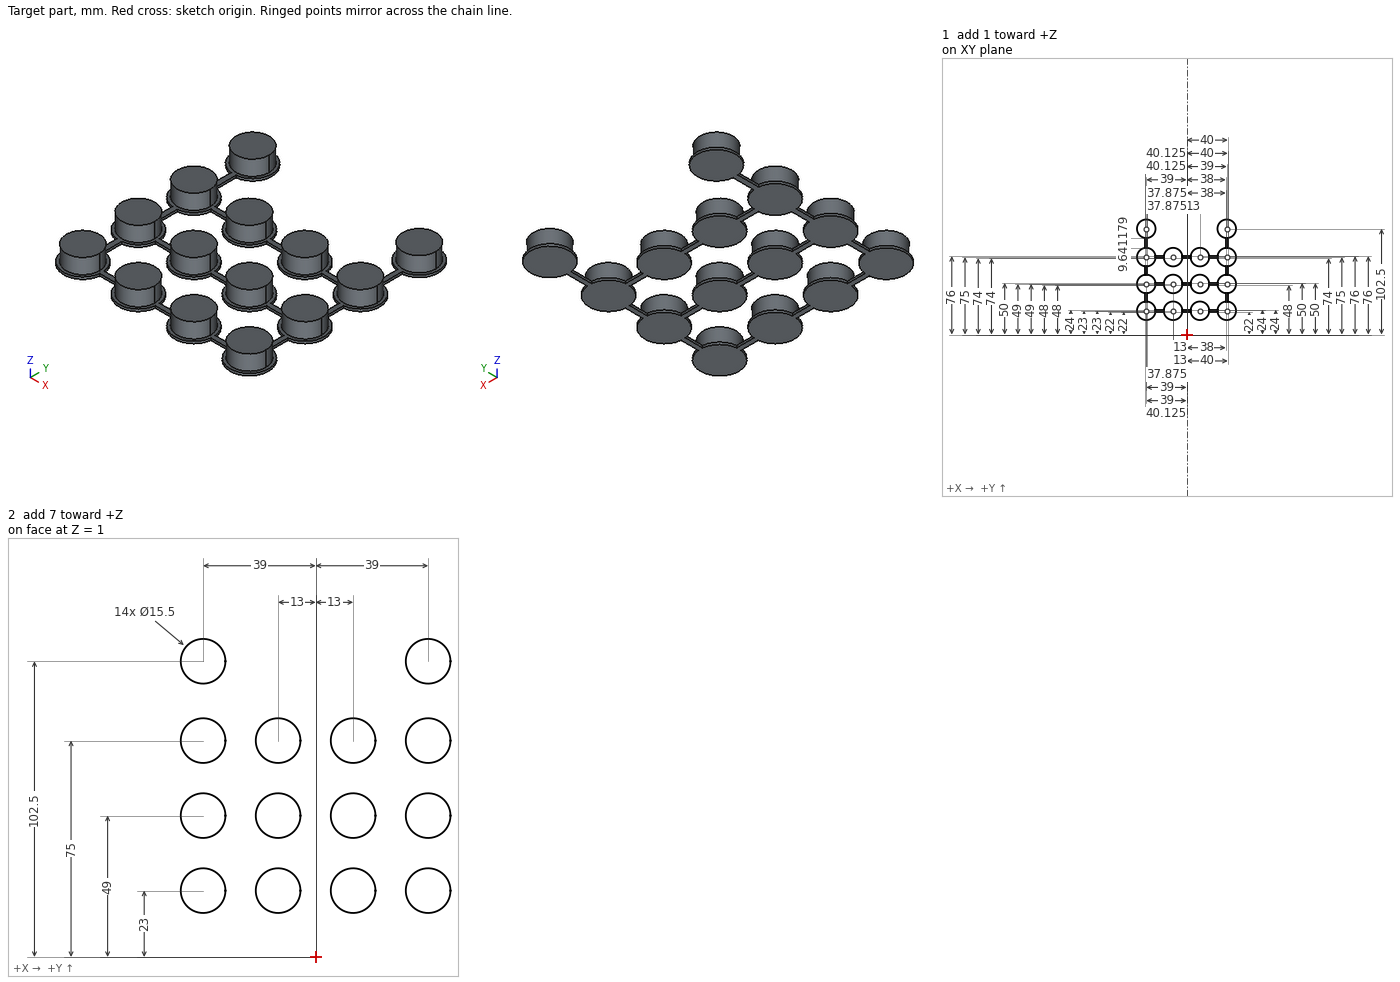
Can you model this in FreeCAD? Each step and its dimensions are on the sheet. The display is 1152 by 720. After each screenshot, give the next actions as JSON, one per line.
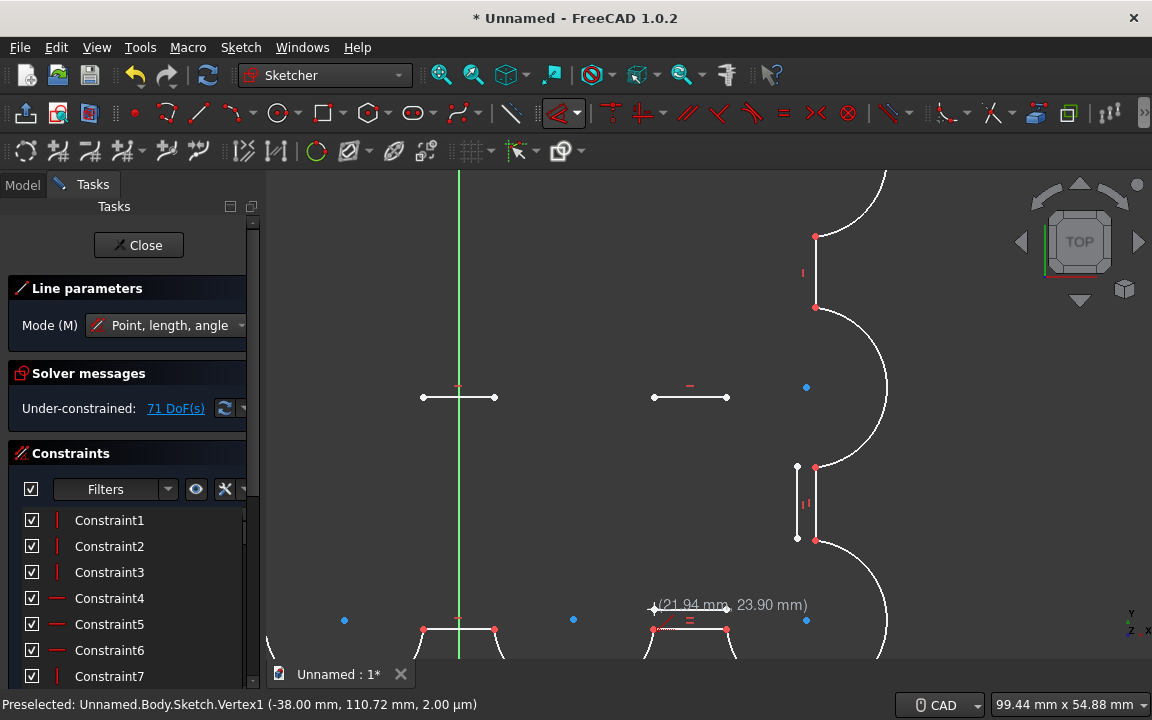
{"action": "left_click", "coordinate": [495, 609]}
{"action": "left_click", "coordinate": [422, 609]}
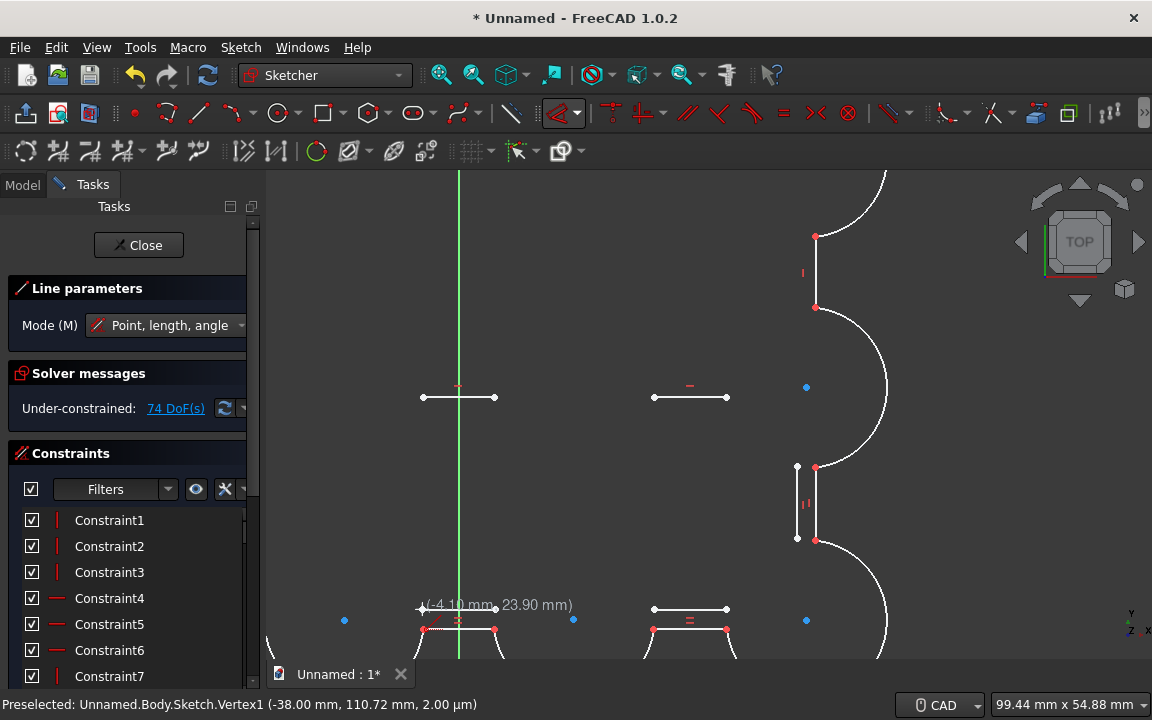
{"action": "scroll", "coordinate": [719, 453], "scroll_direction": "down", "scroll_amount": 6}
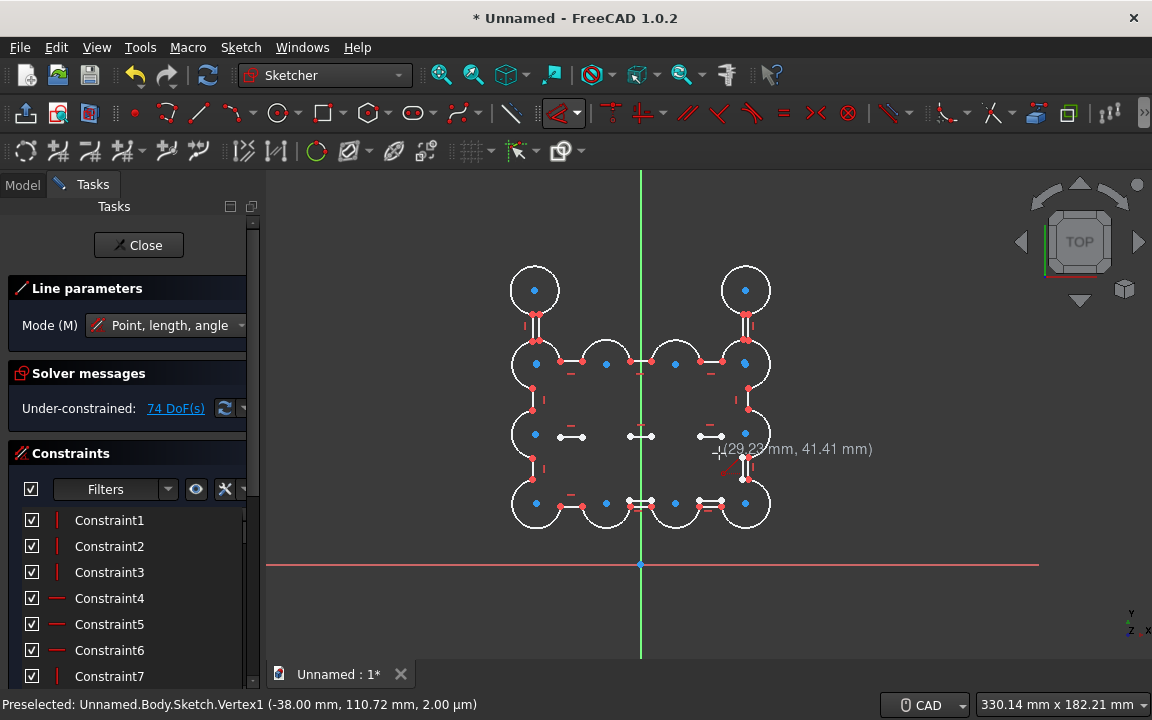
{"action": "scroll", "coordinate": [582, 500], "scroll_direction": "up", "scroll_amount": 6}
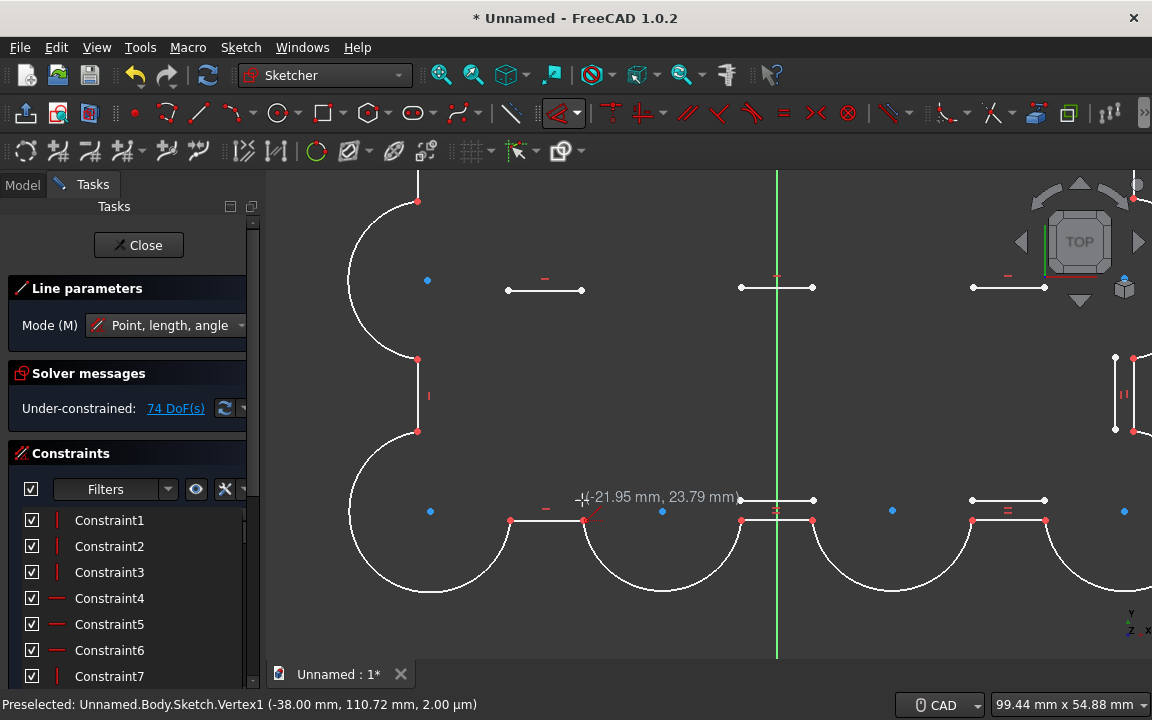
{"action": "left_click", "coordinate": [581, 500]}
{"action": "left_click", "coordinate": [509, 500]}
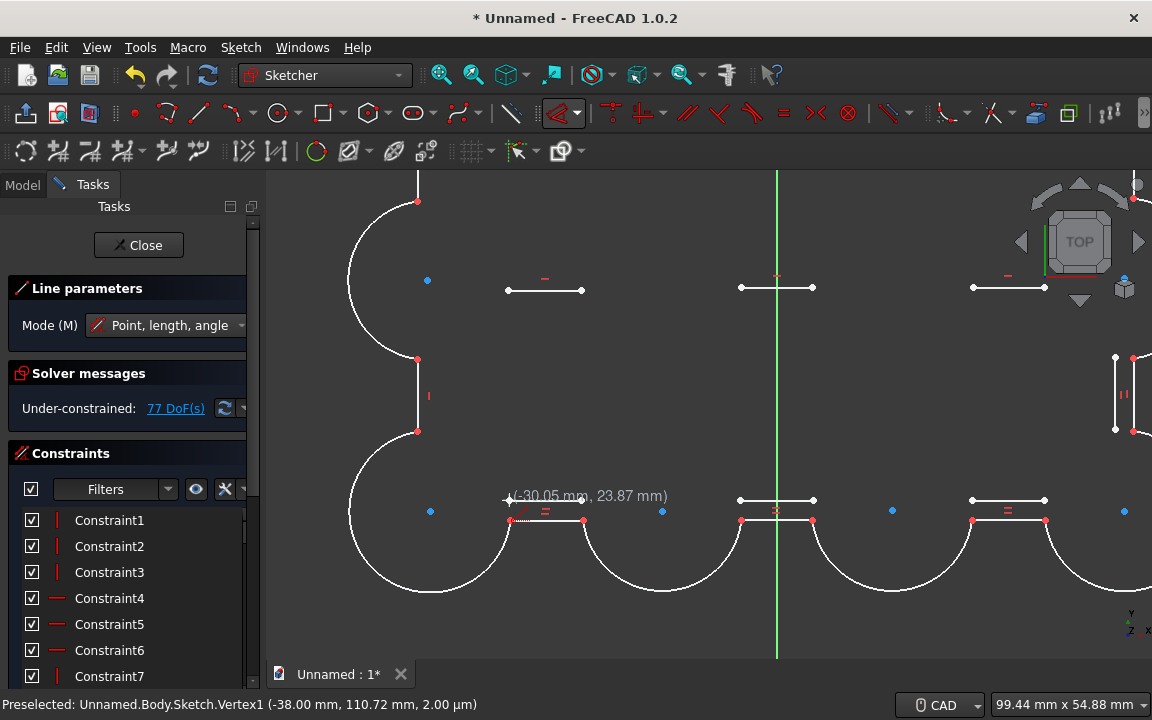
{"action": "left_click", "coordinate": [439, 429]}
{"action": "left_click", "coordinate": [439, 357]}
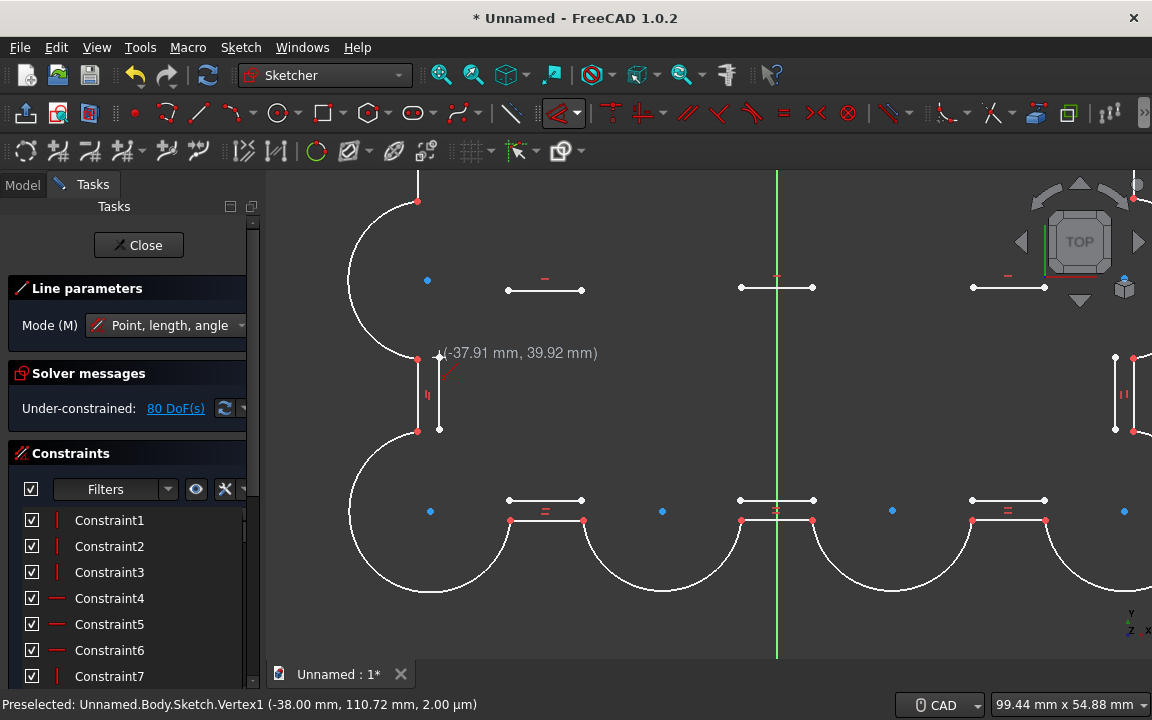
{"action": "left_click", "coordinate": [232, 114]}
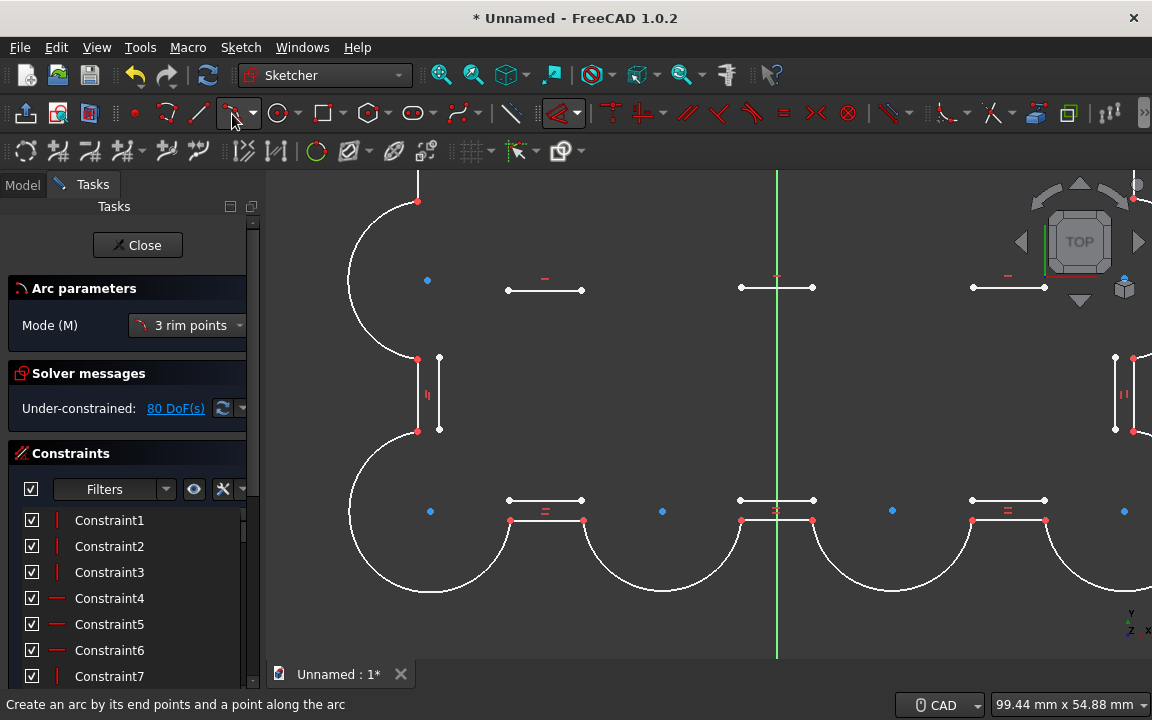
{"action": "left_click", "coordinate": [582, 291]}
{"action": "left_click", "coordinate": [742, 288]}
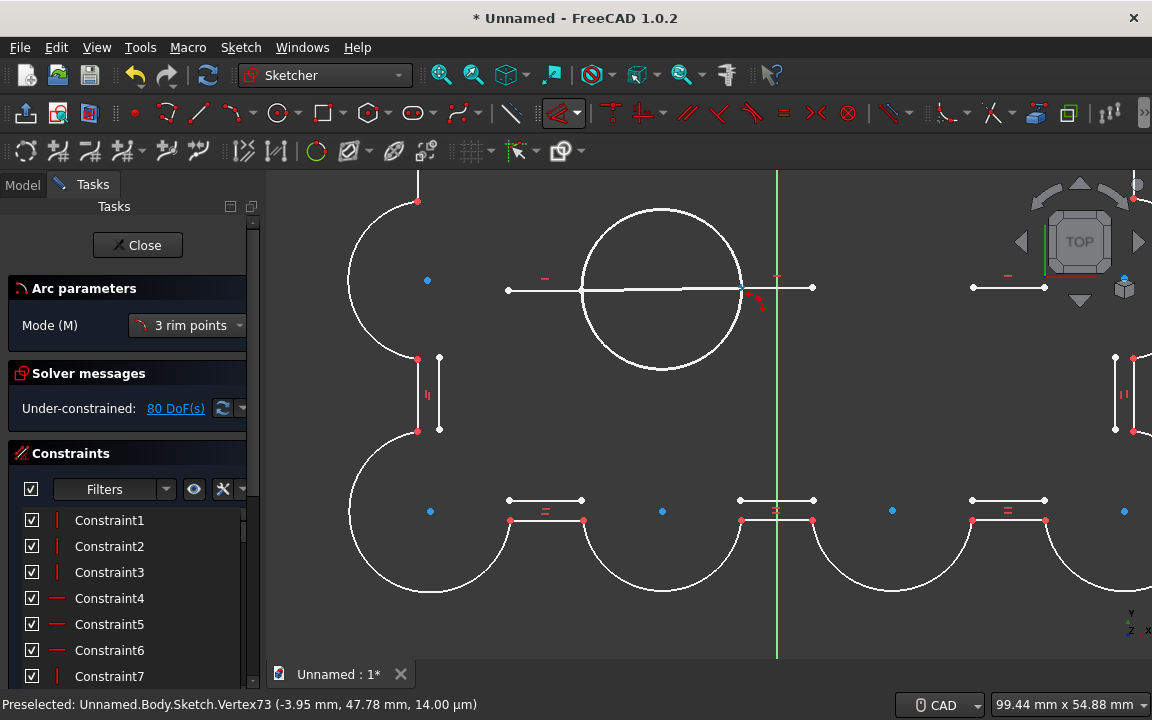
{"action": "scroll", "coordinate": [582, 500], "scroll_direction": "down", "scroll_amount": 6}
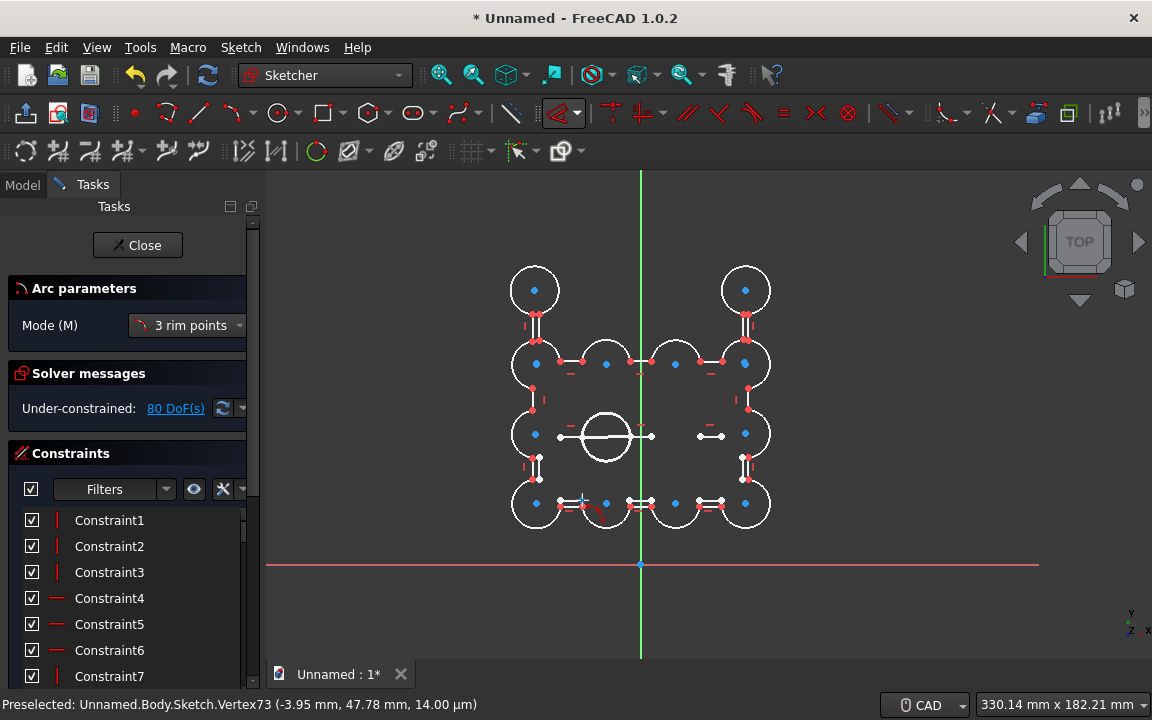
{"action": "left_click", "coordinate": [606, 457]}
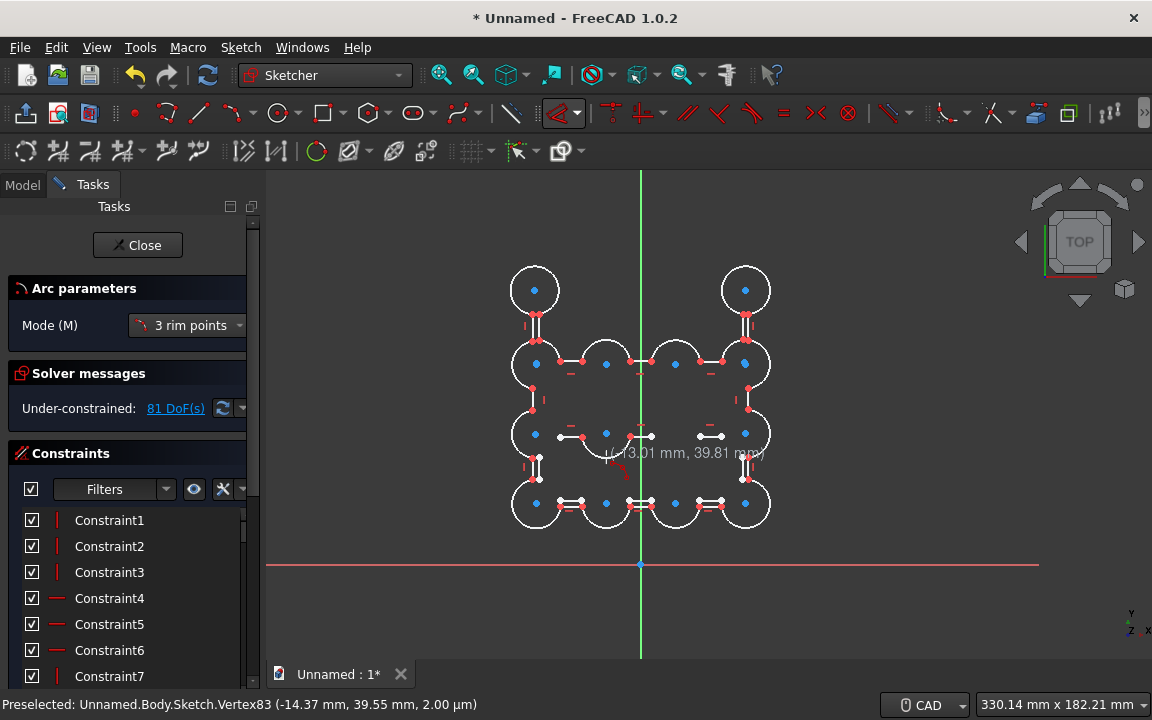
{"action": "scroll", "coordinate": [652, 436], "scroll_direction": "up", "scroll_amount": 2}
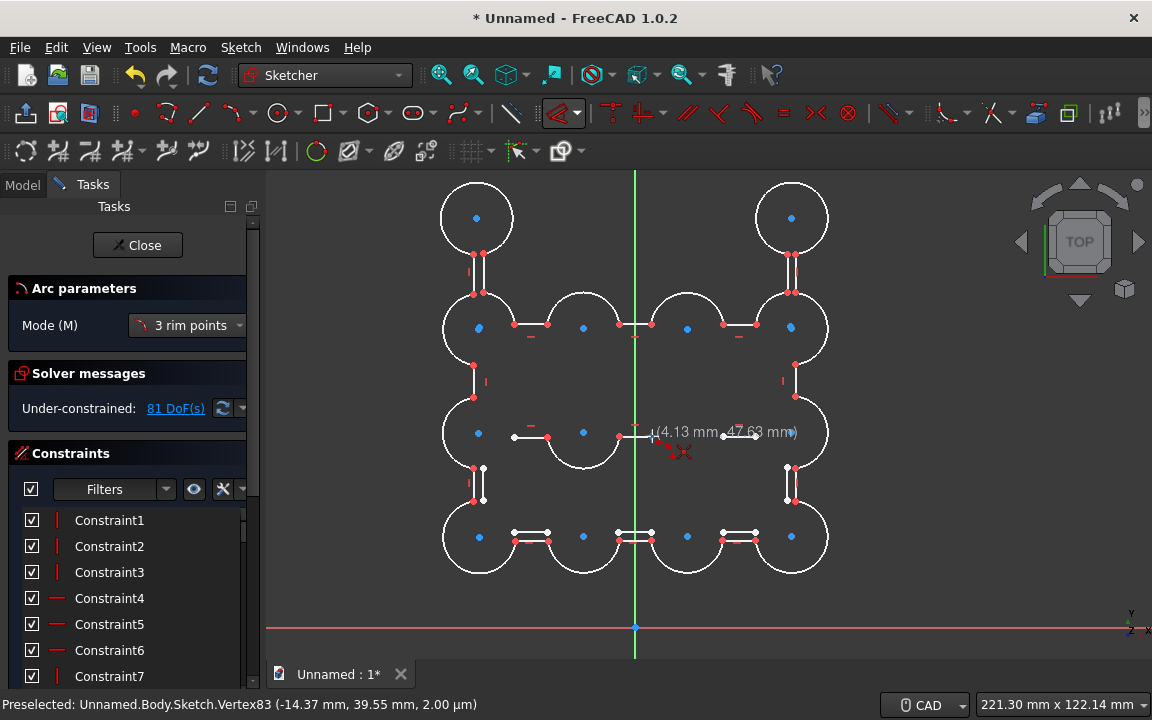
{"action": "left_click", "coordinate": [651, 437]}
{"action": "left_click", "coordinate": [723, 437]}
{"action": "left_click", "coordinate": [687, 468]}